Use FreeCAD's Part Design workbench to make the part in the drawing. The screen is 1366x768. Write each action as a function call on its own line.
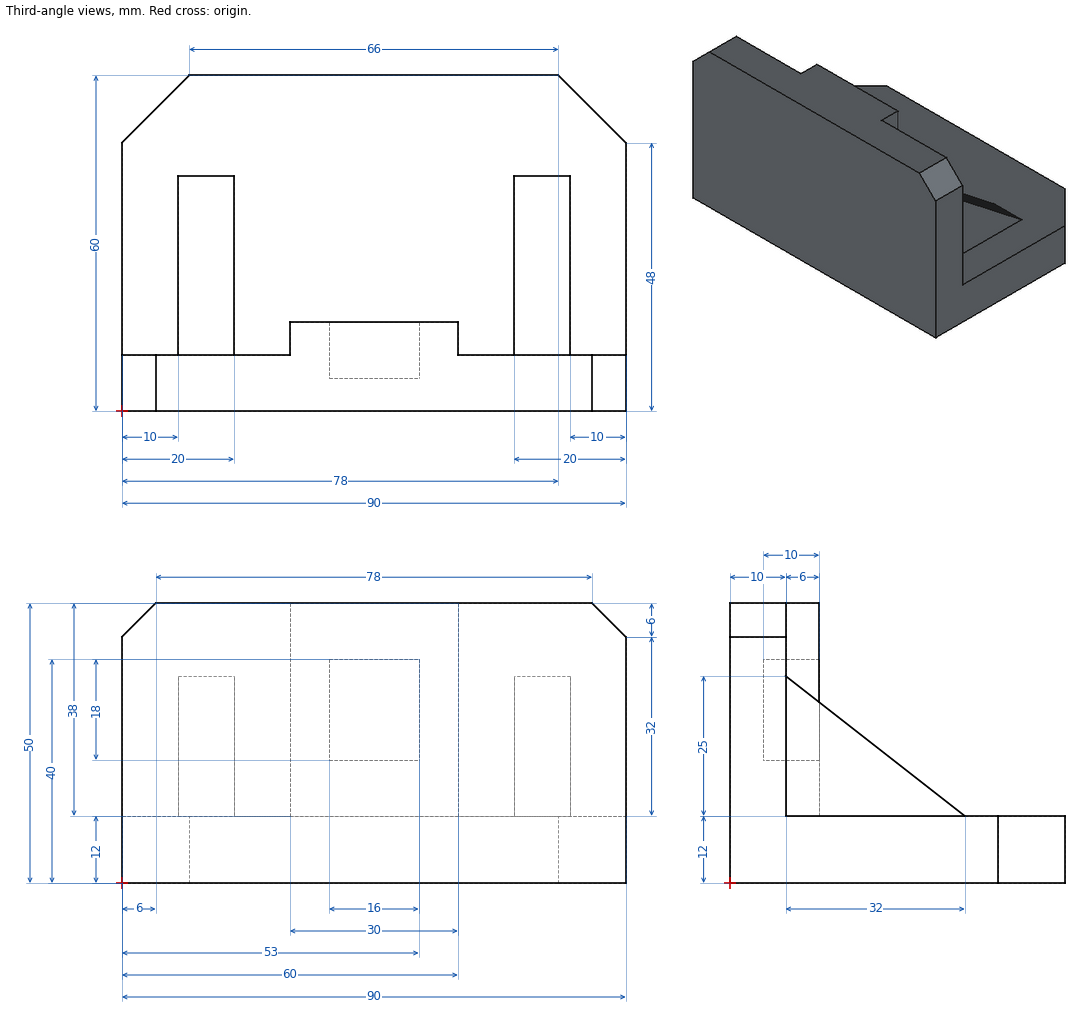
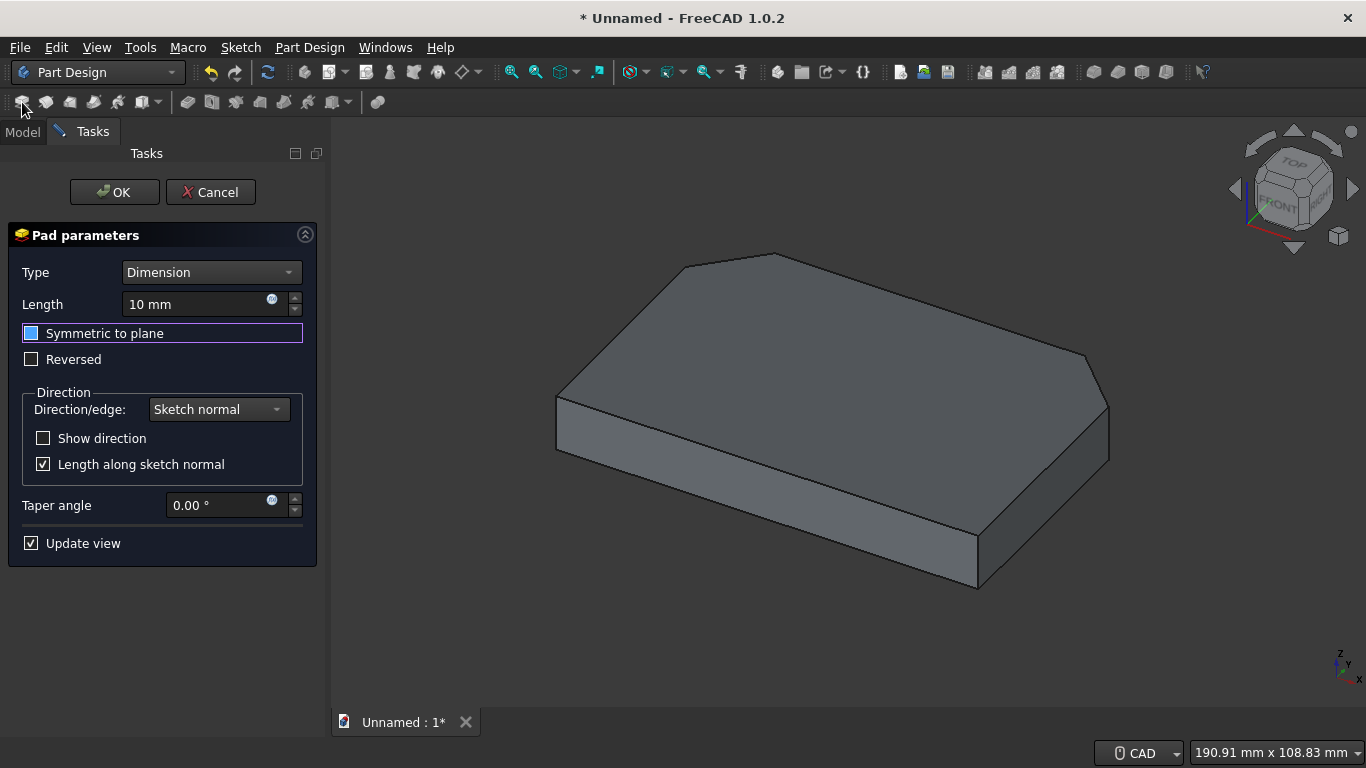
click(30, 359)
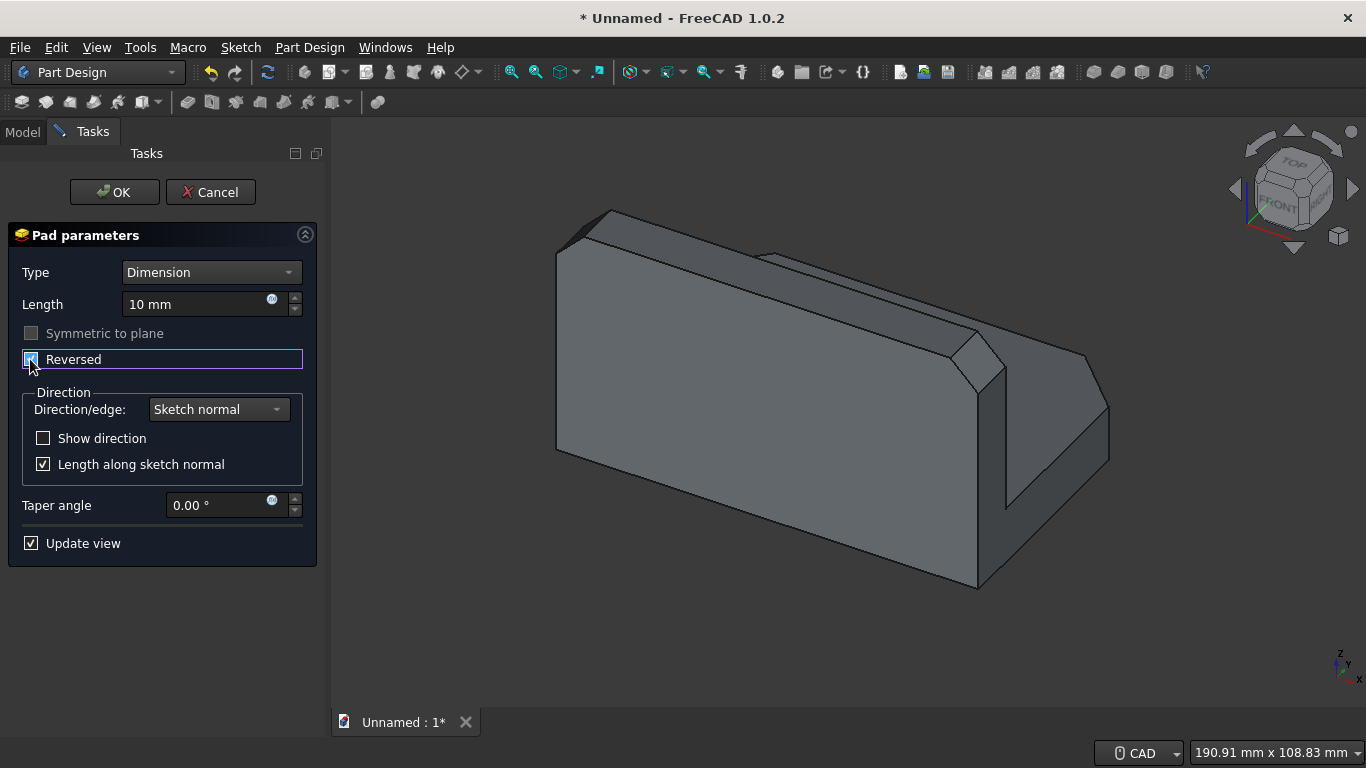
click(115, 192)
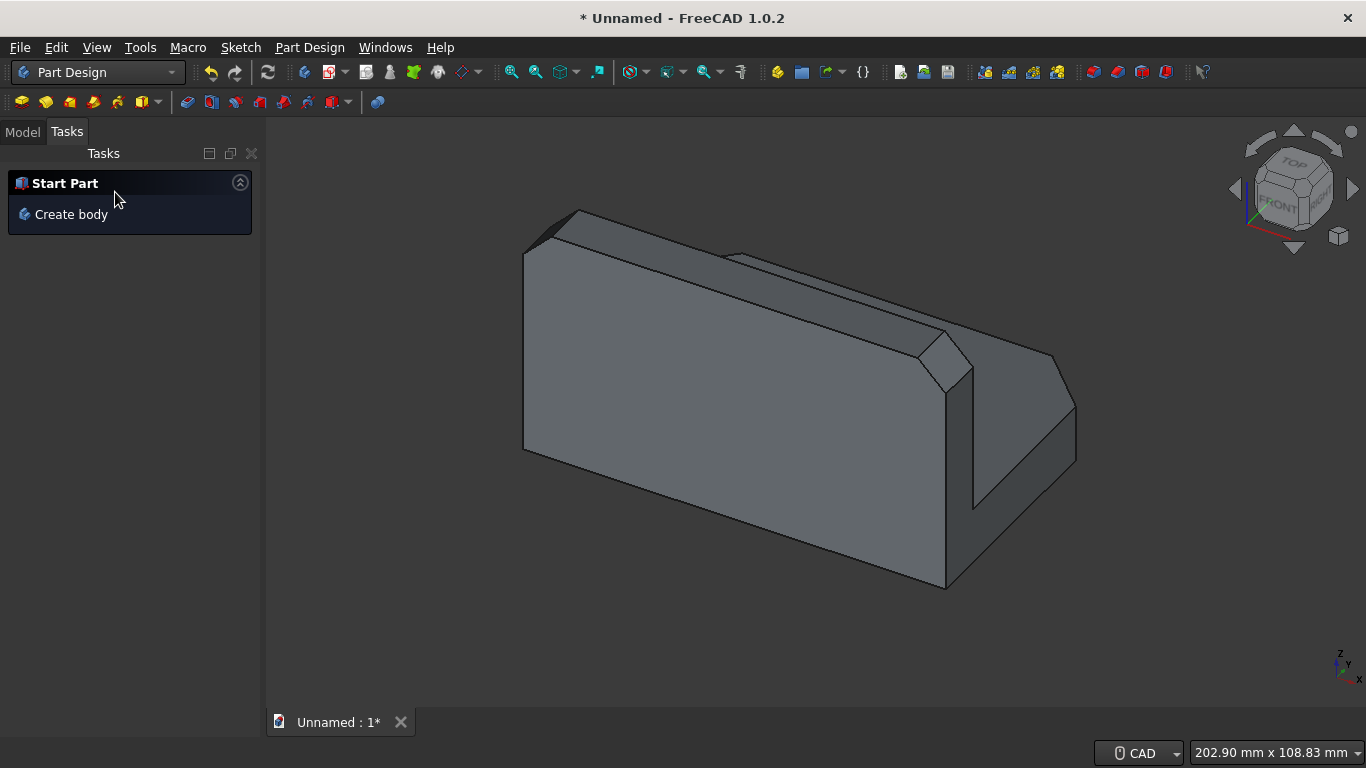
click(512, 72)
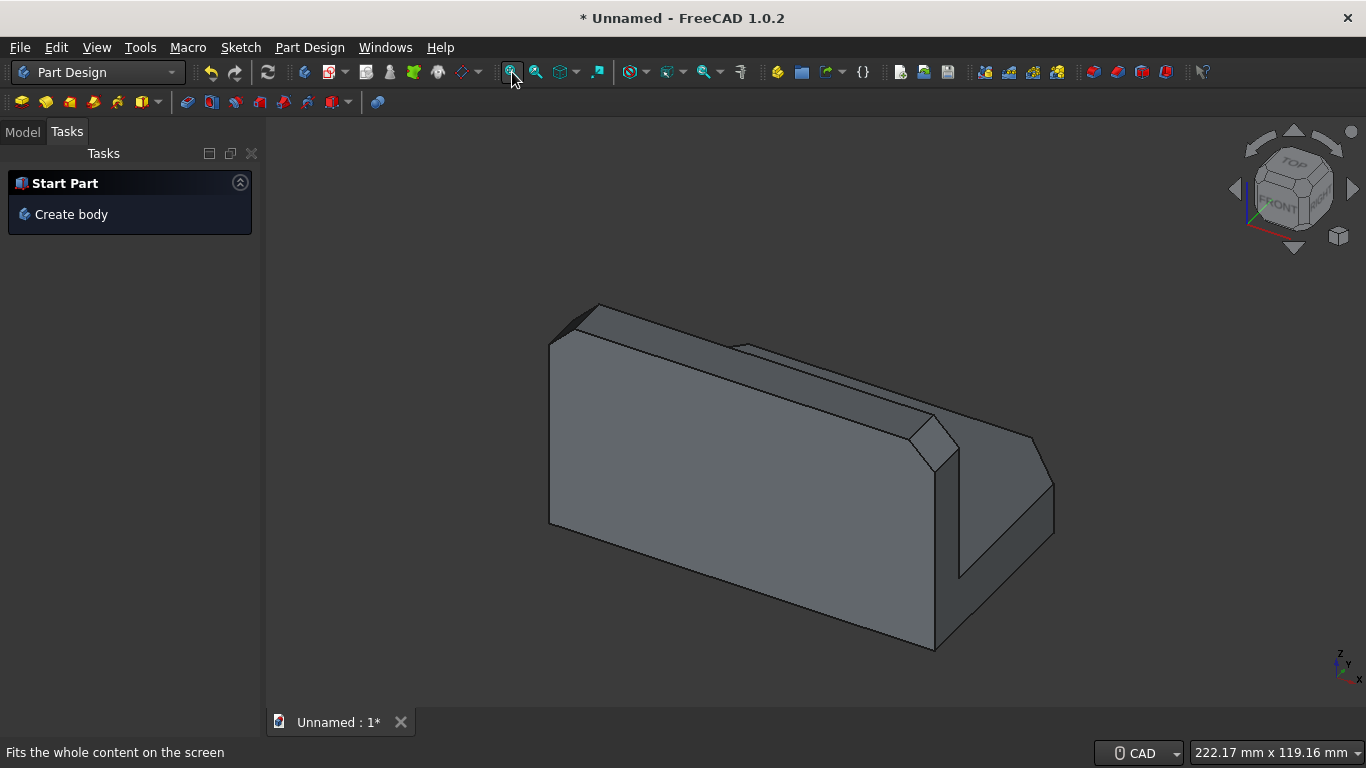
key(4)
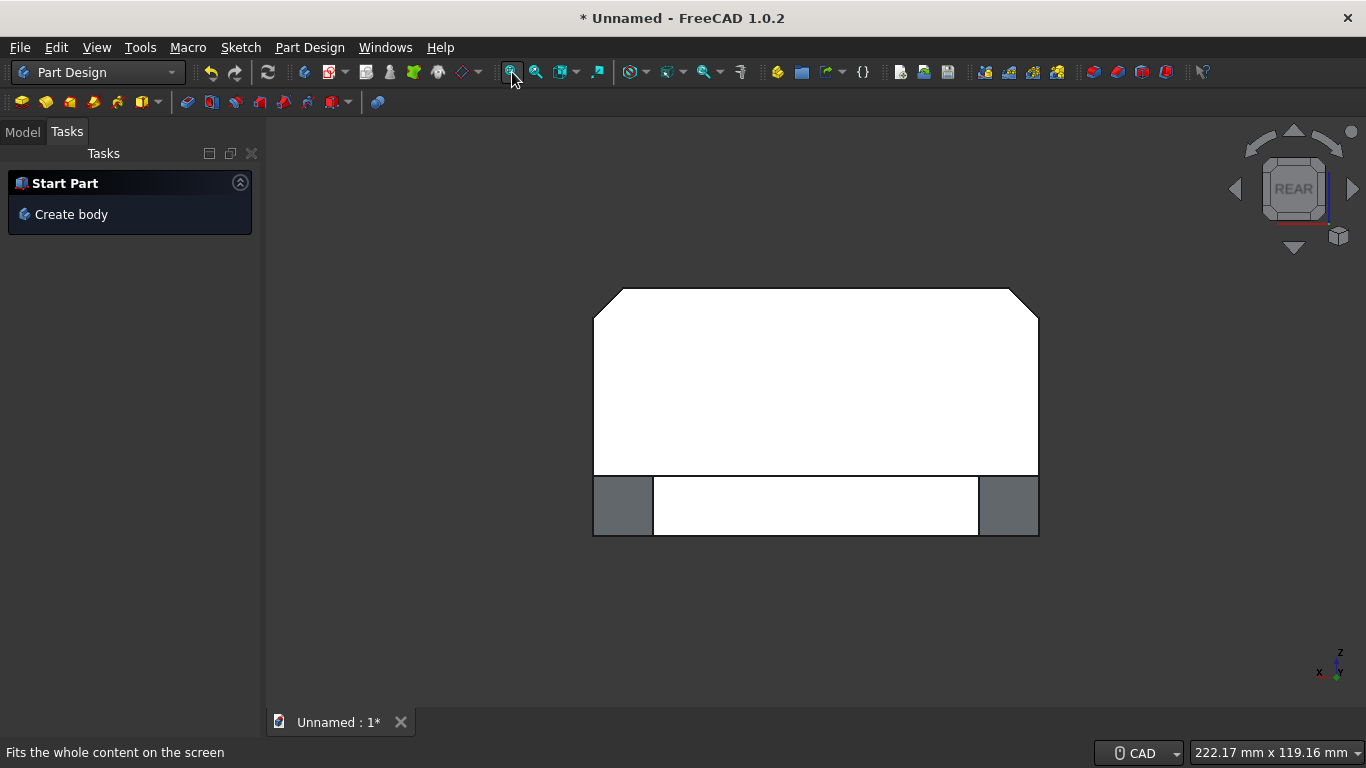
click(512, 72)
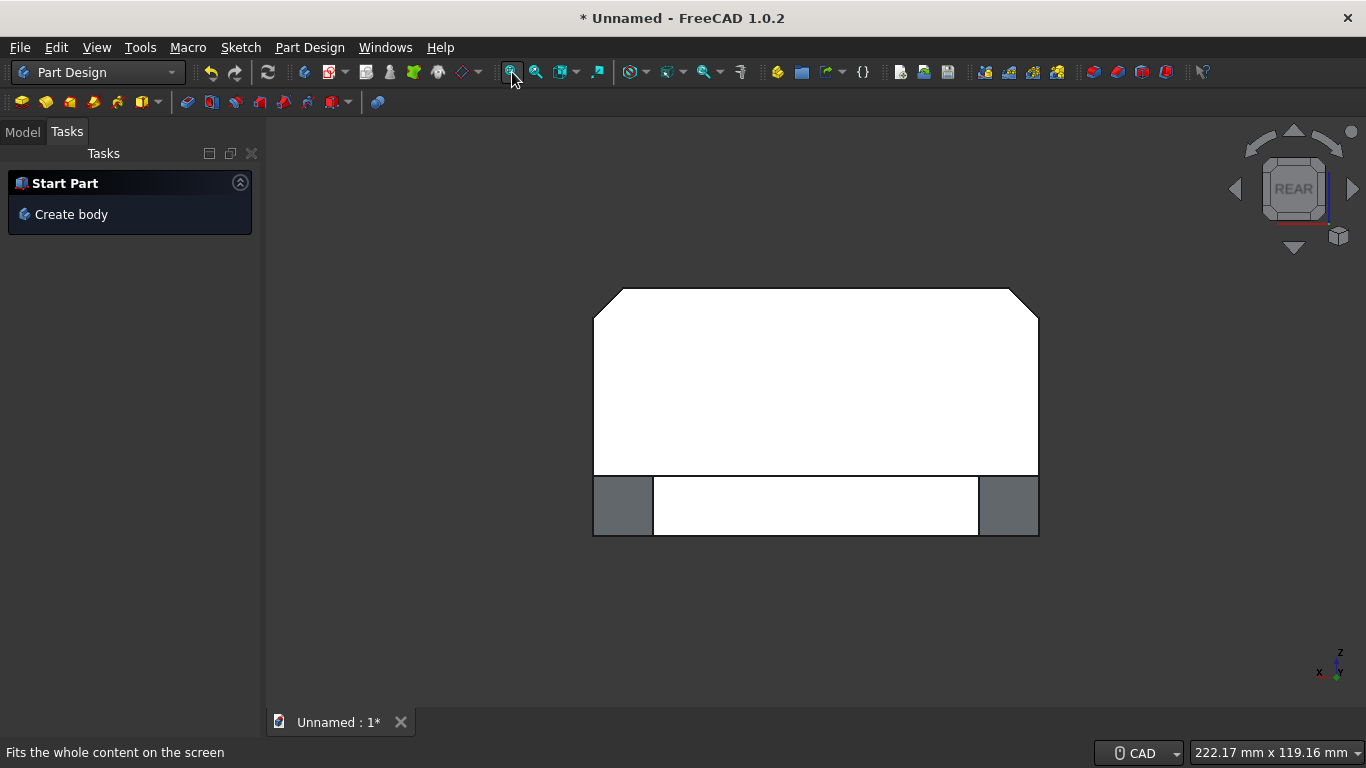
click(689, 381)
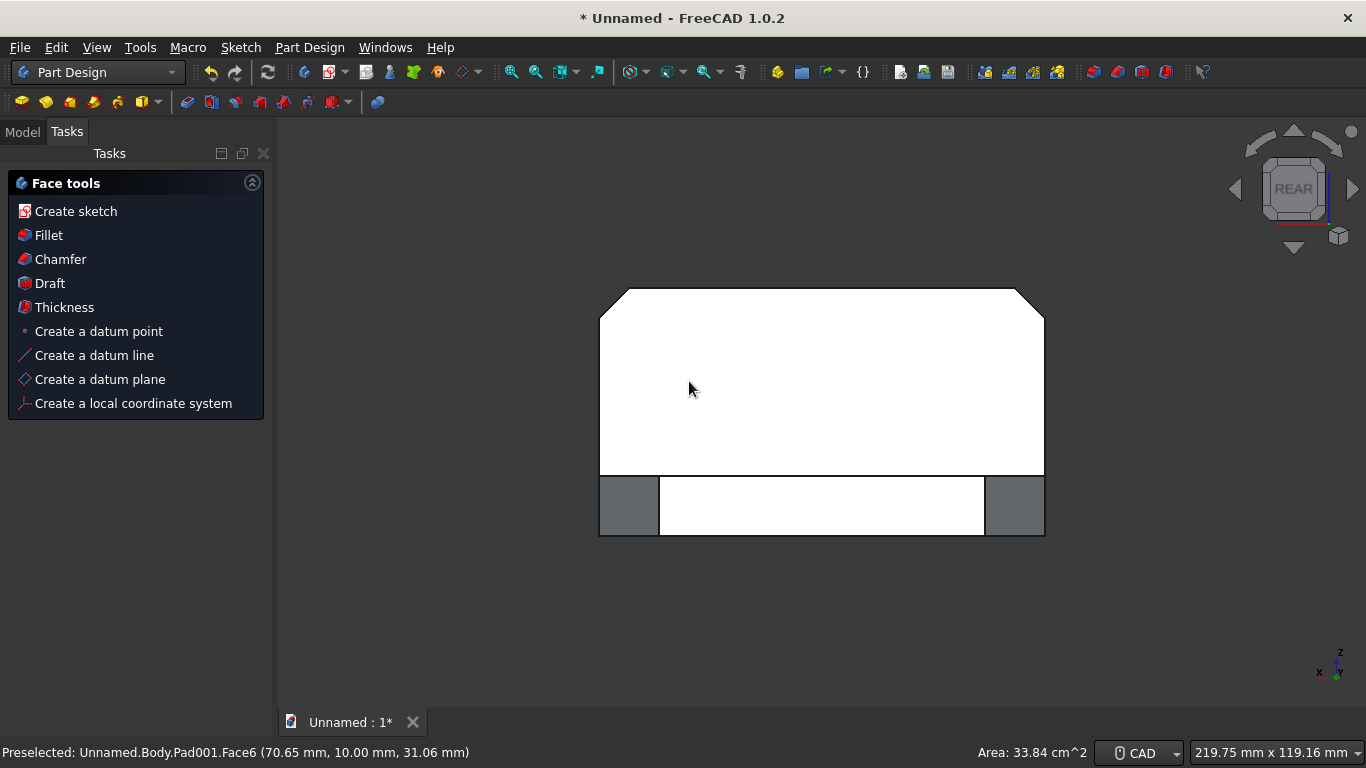
click(330, 72)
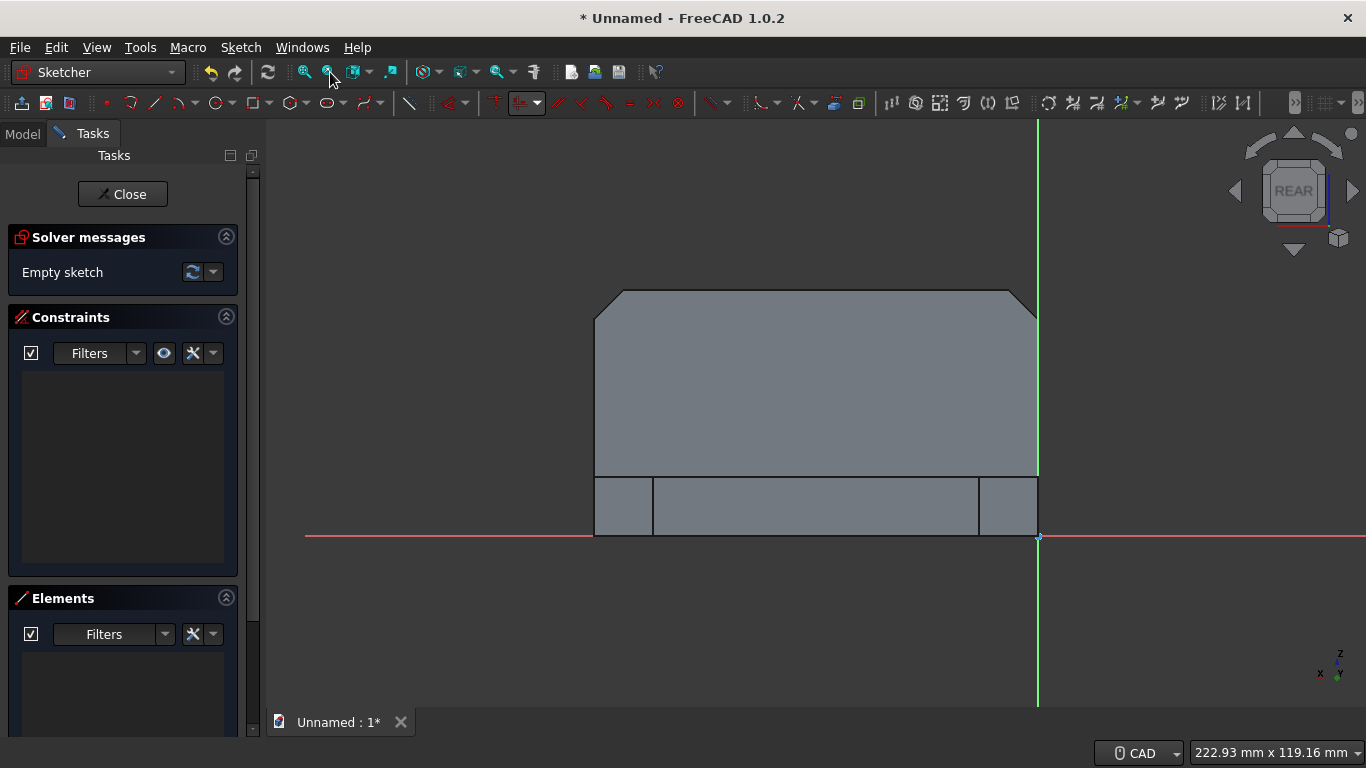
scroll(1180, 413, up, 2)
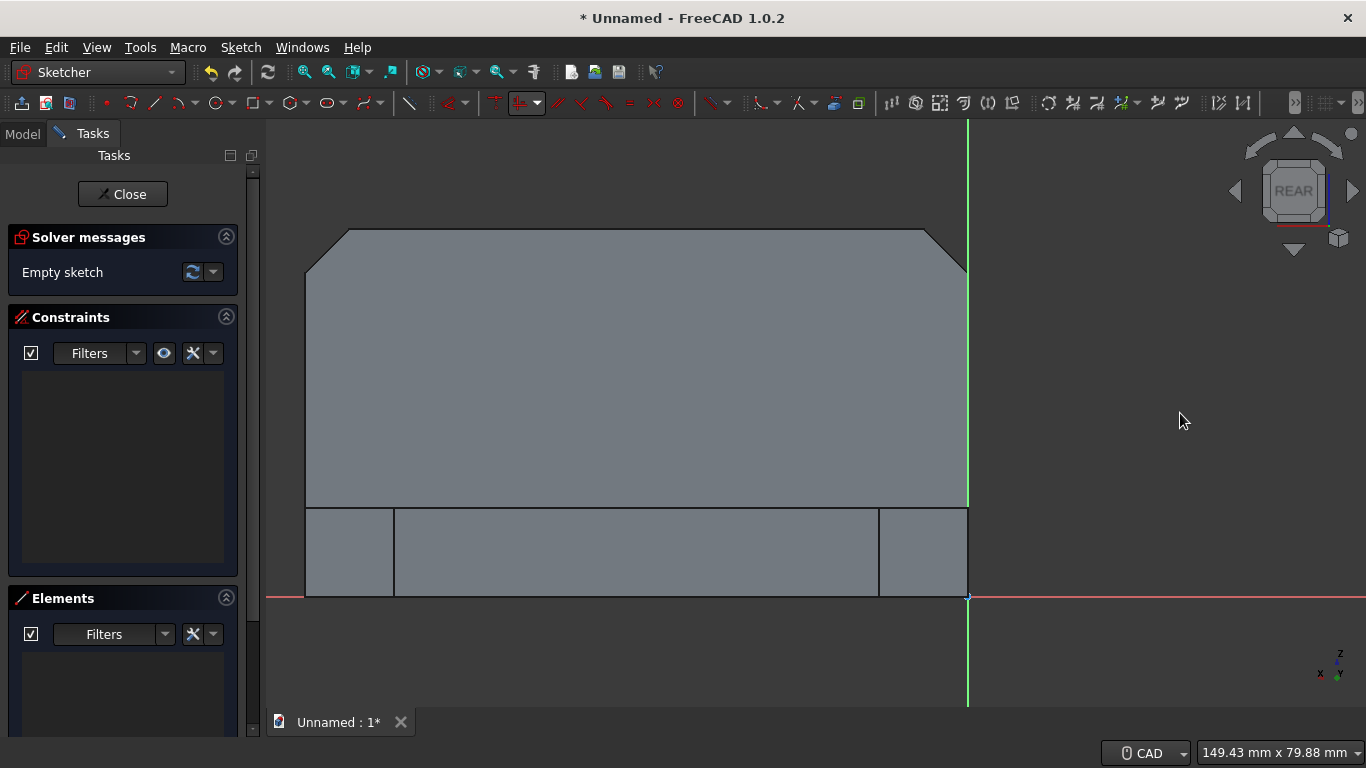
click(254, 104)